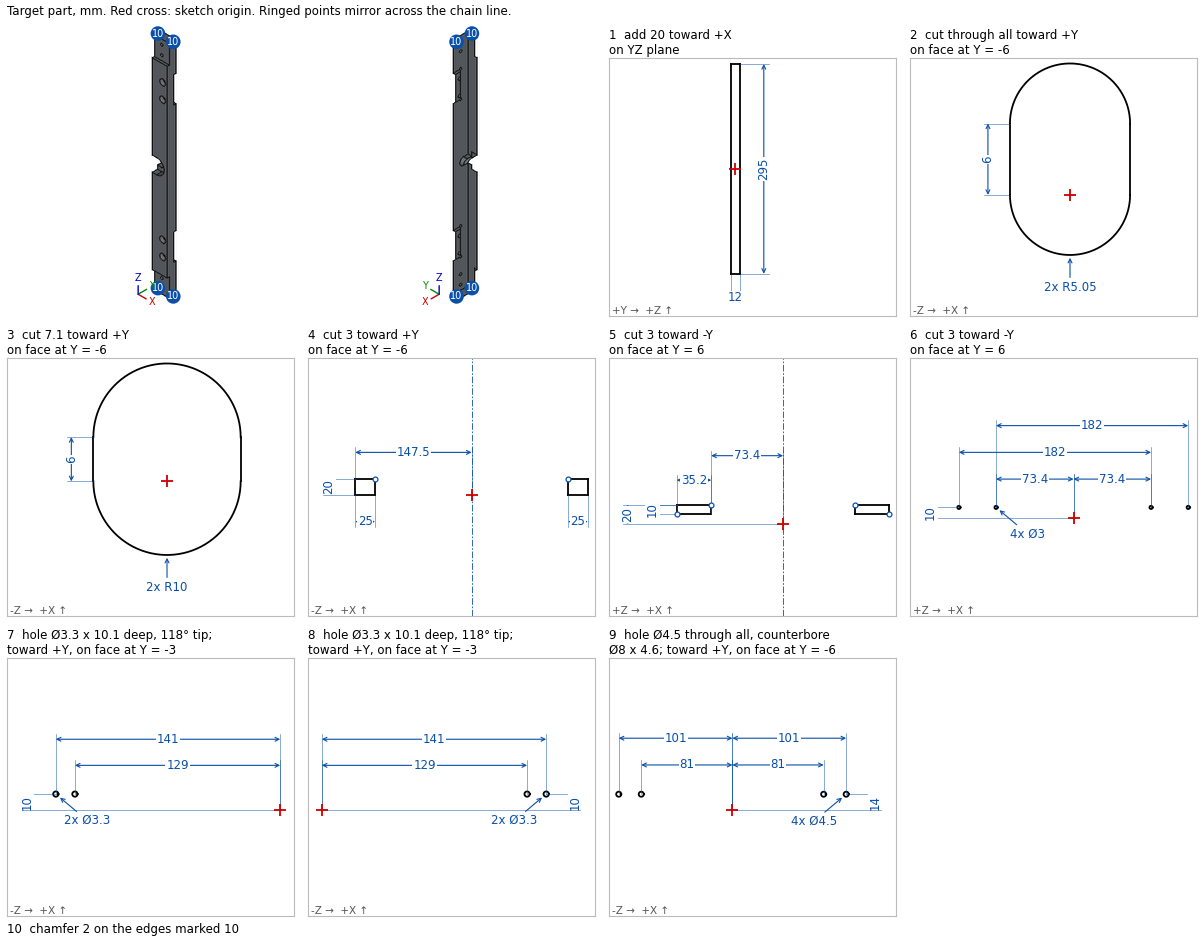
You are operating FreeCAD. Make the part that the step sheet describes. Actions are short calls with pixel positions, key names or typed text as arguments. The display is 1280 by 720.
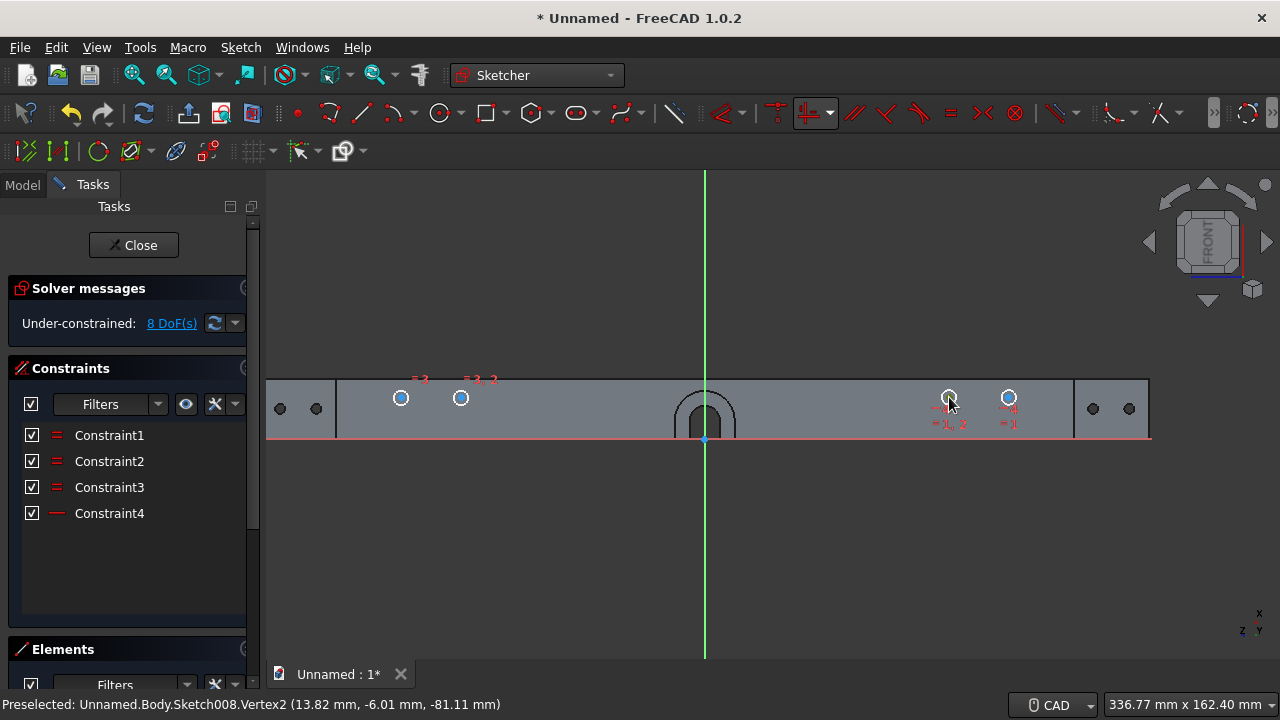
click(461, 398)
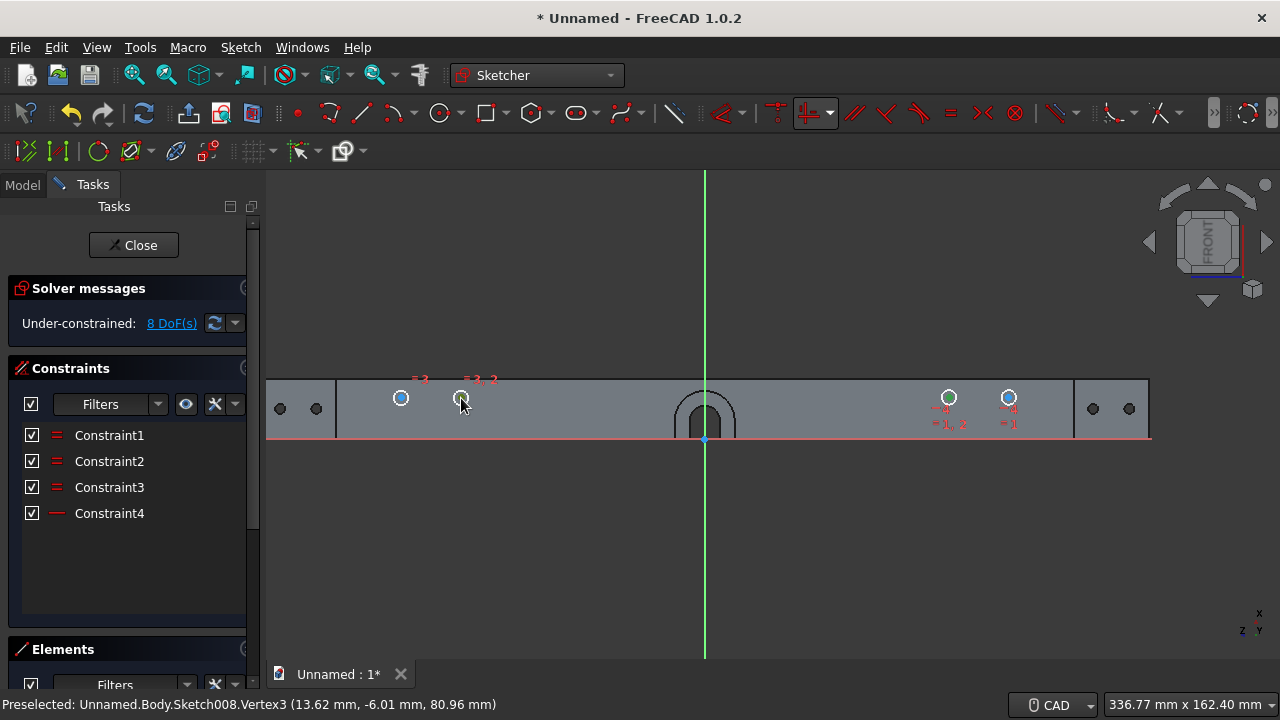
click(832, 114)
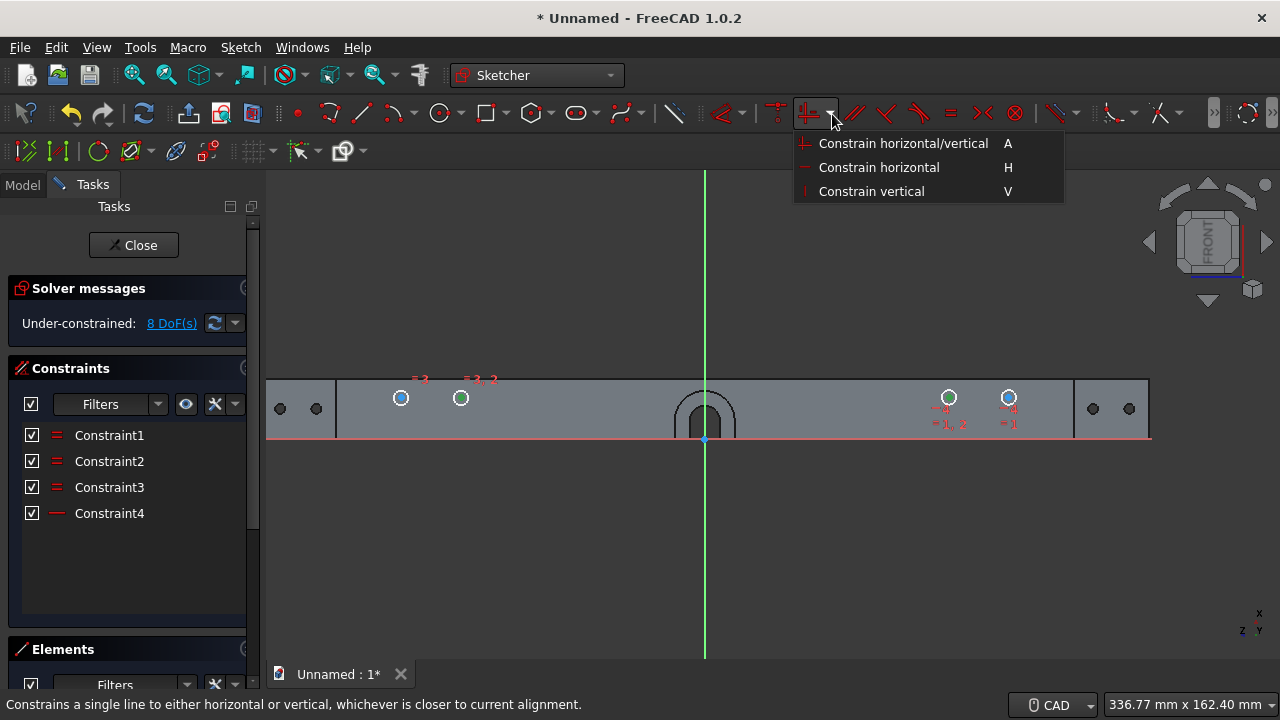
click(929, 167)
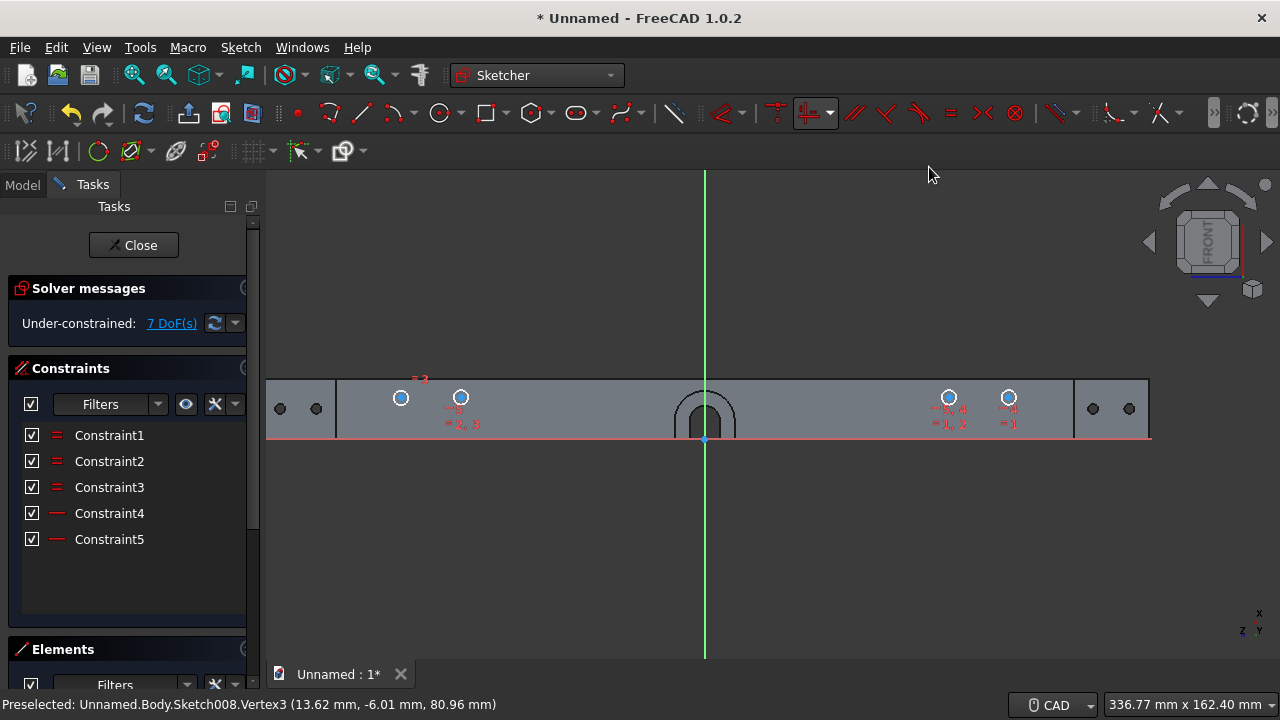
click(461, 397)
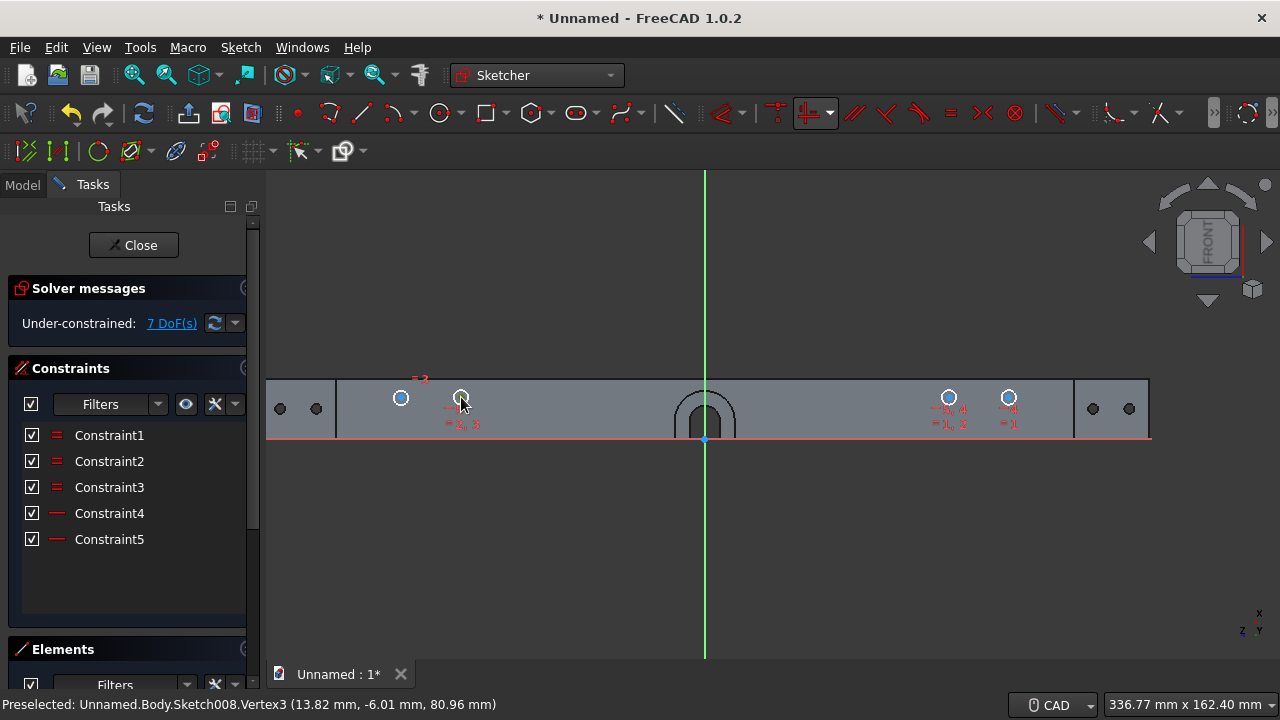
click(401, 398)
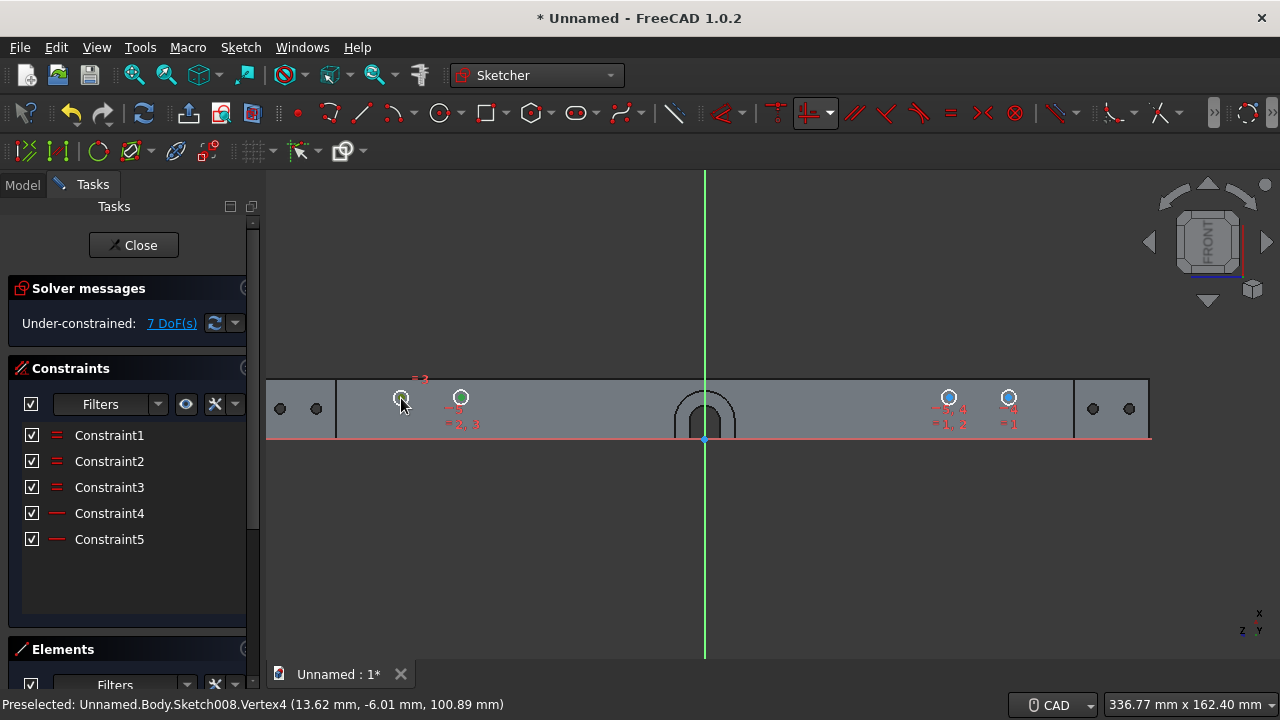
key(h)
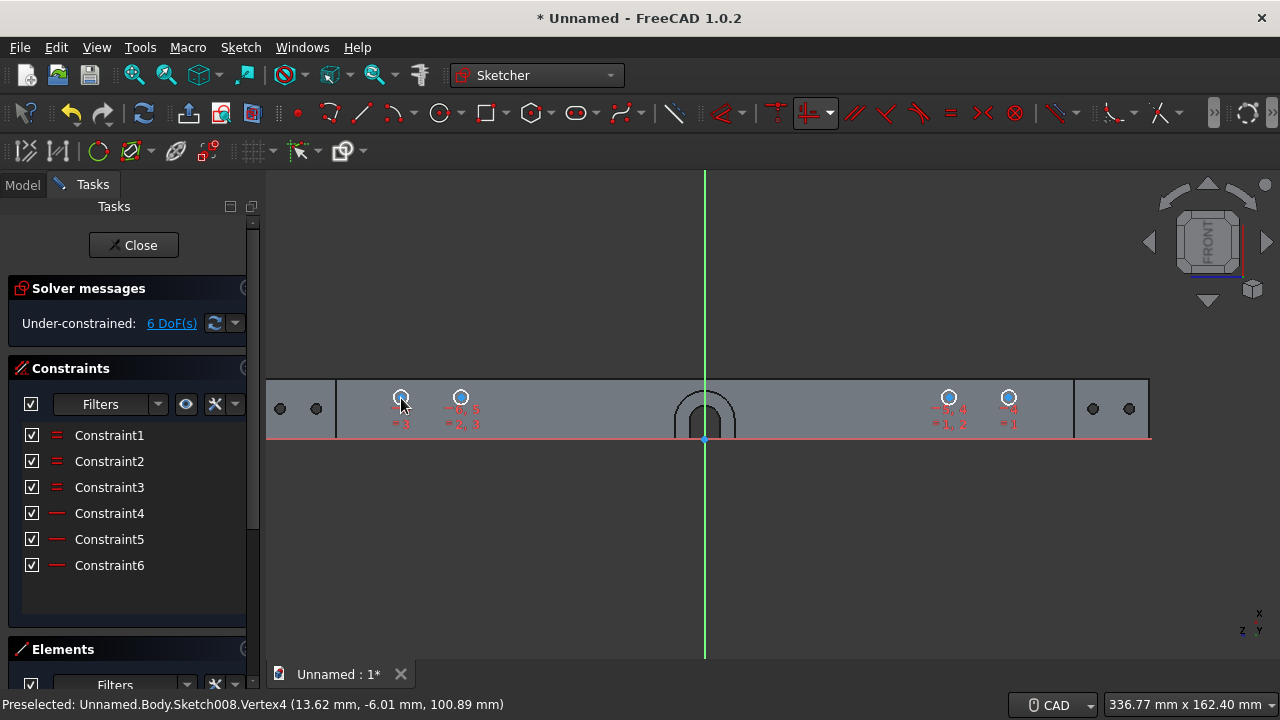
click(722, 114)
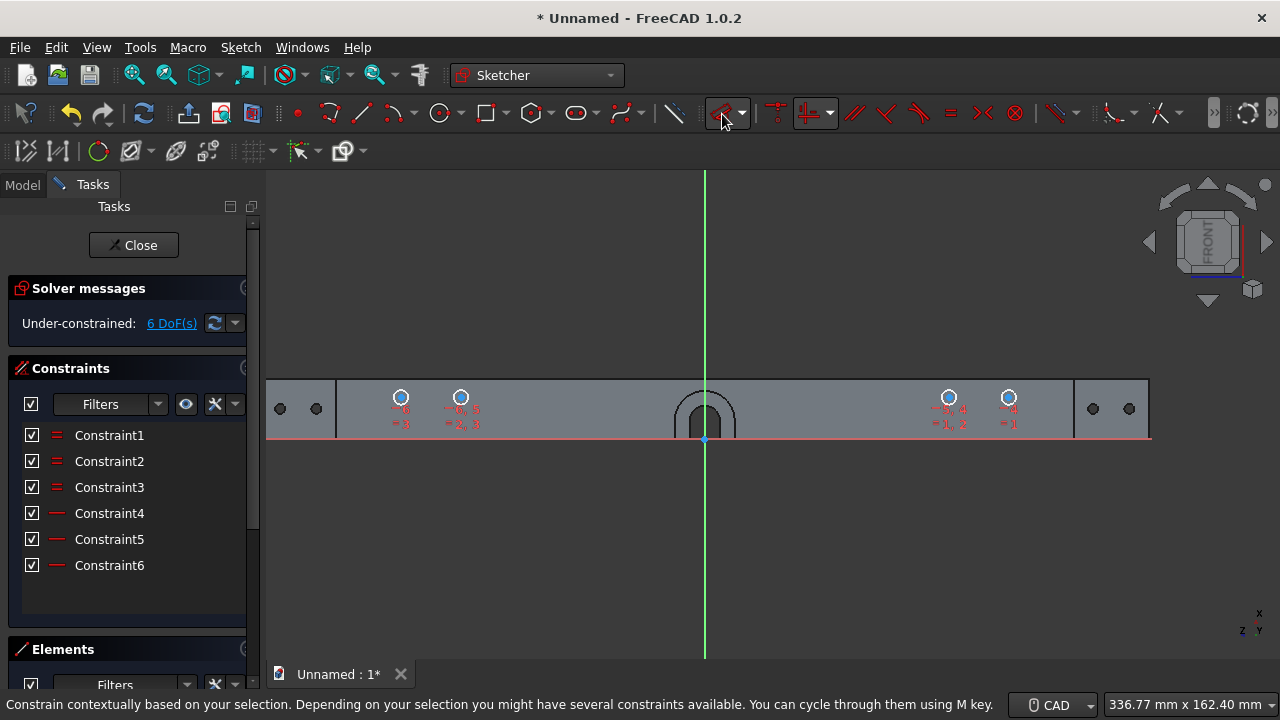
scroll(1004, 392, up, 6)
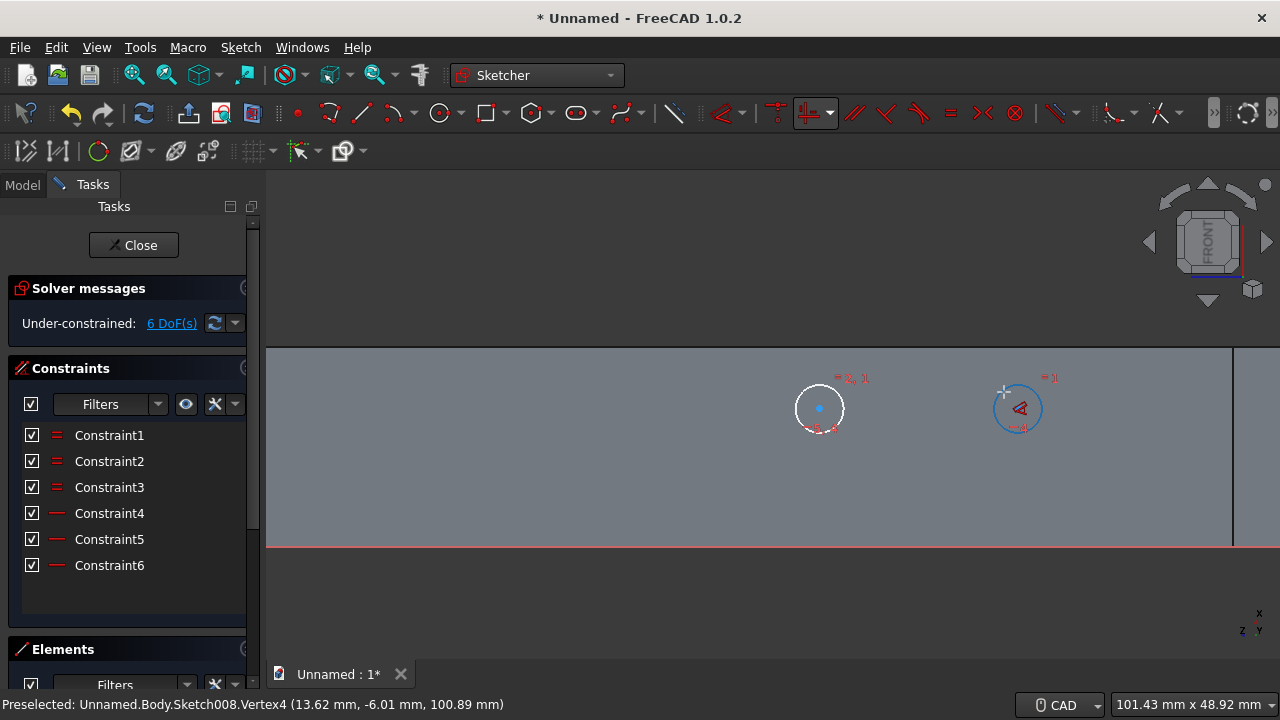
click(1001, 392)
click(978, 369)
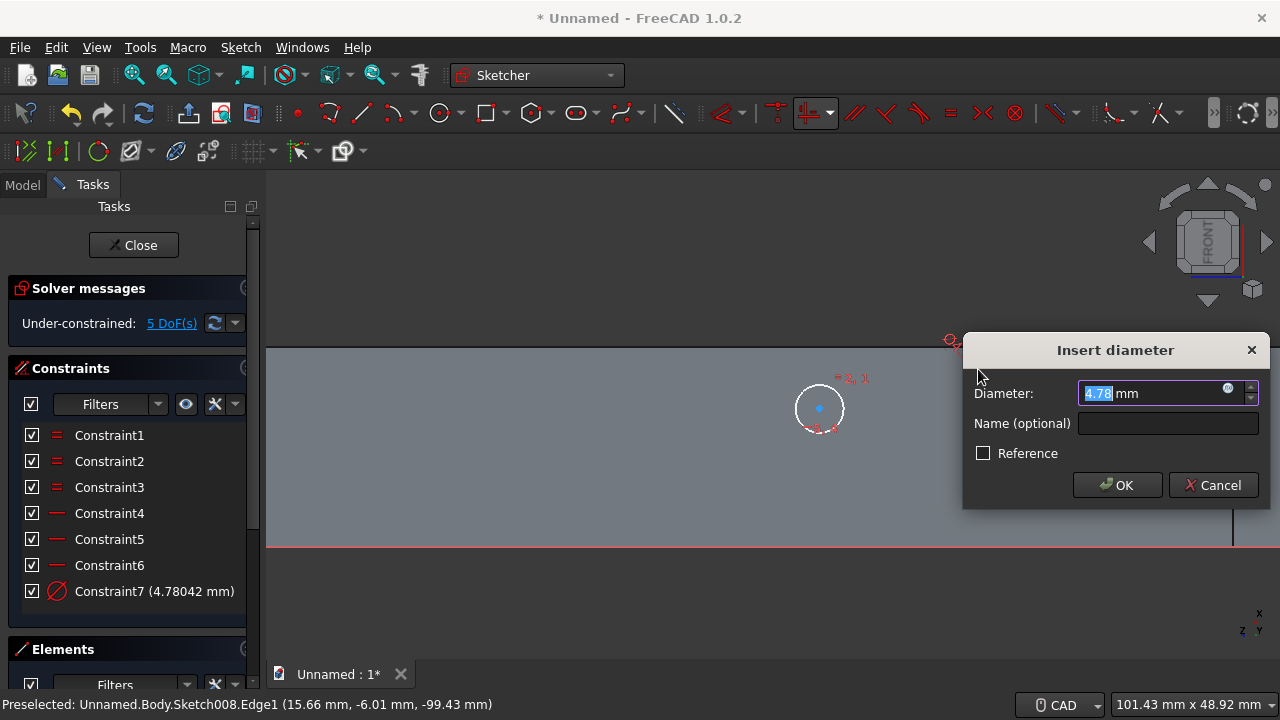
text(4.5)
key(Return)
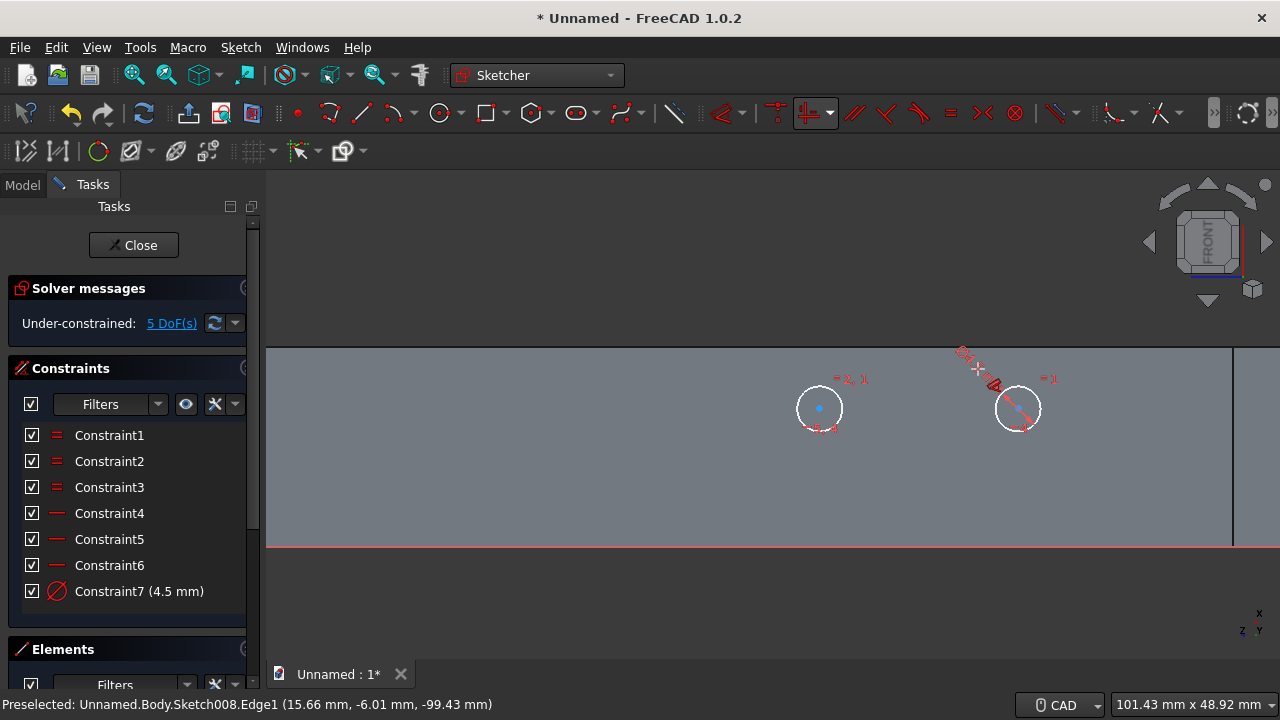
click(1018, 409)
click(1052, 478)